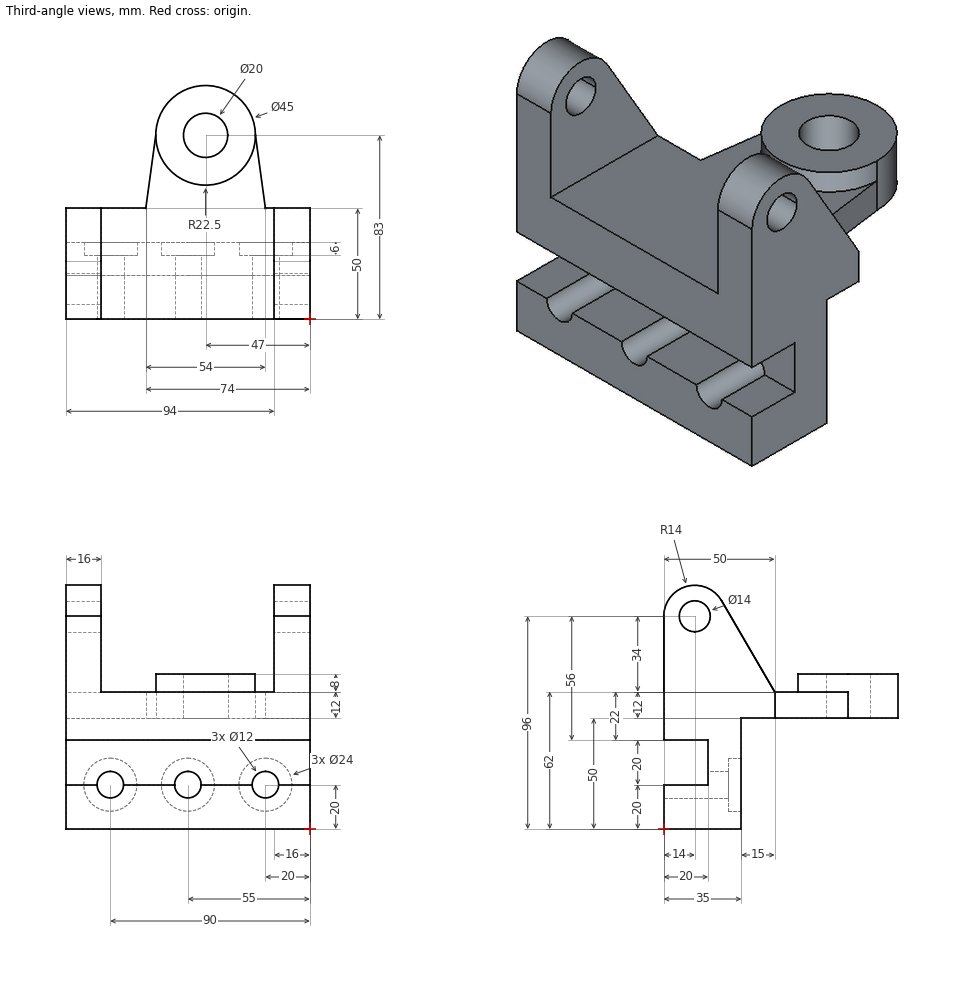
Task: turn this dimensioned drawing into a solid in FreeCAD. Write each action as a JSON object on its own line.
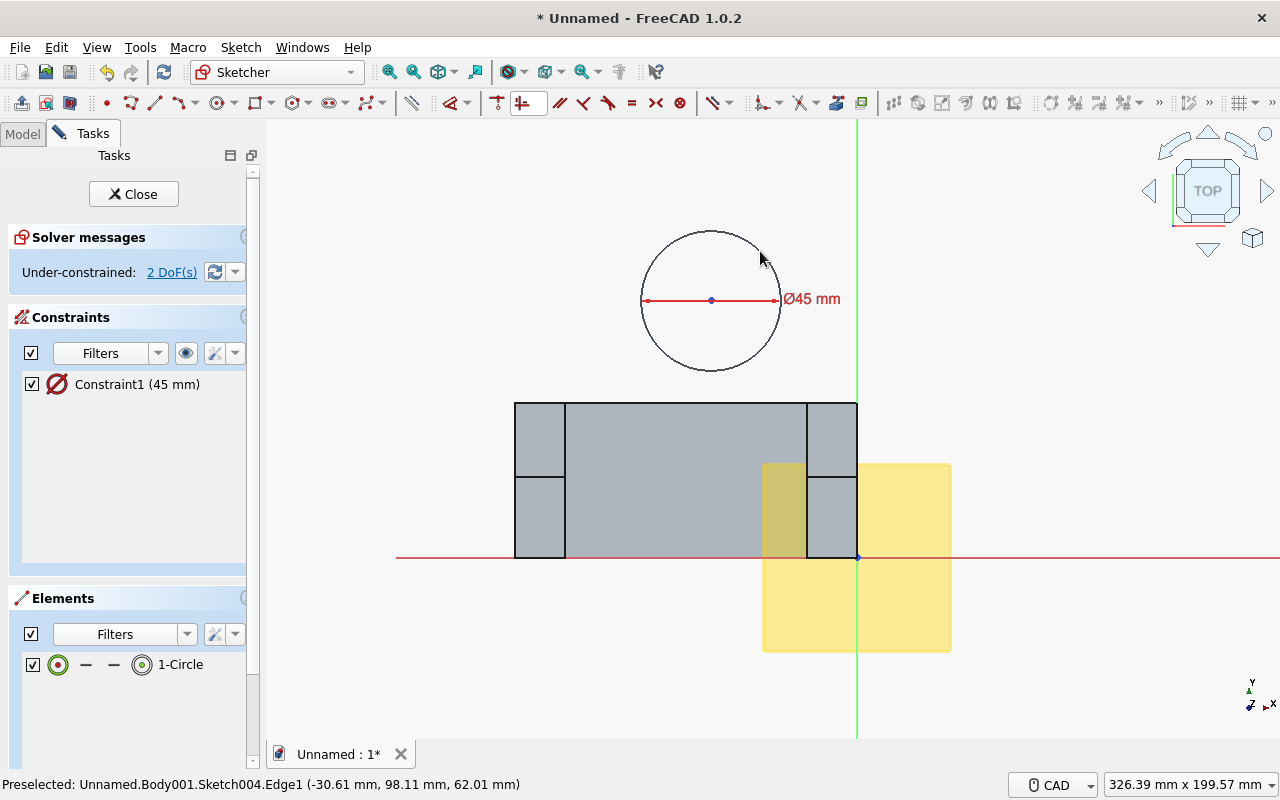
{"action": "left_click", "coordinate": [450, 104]}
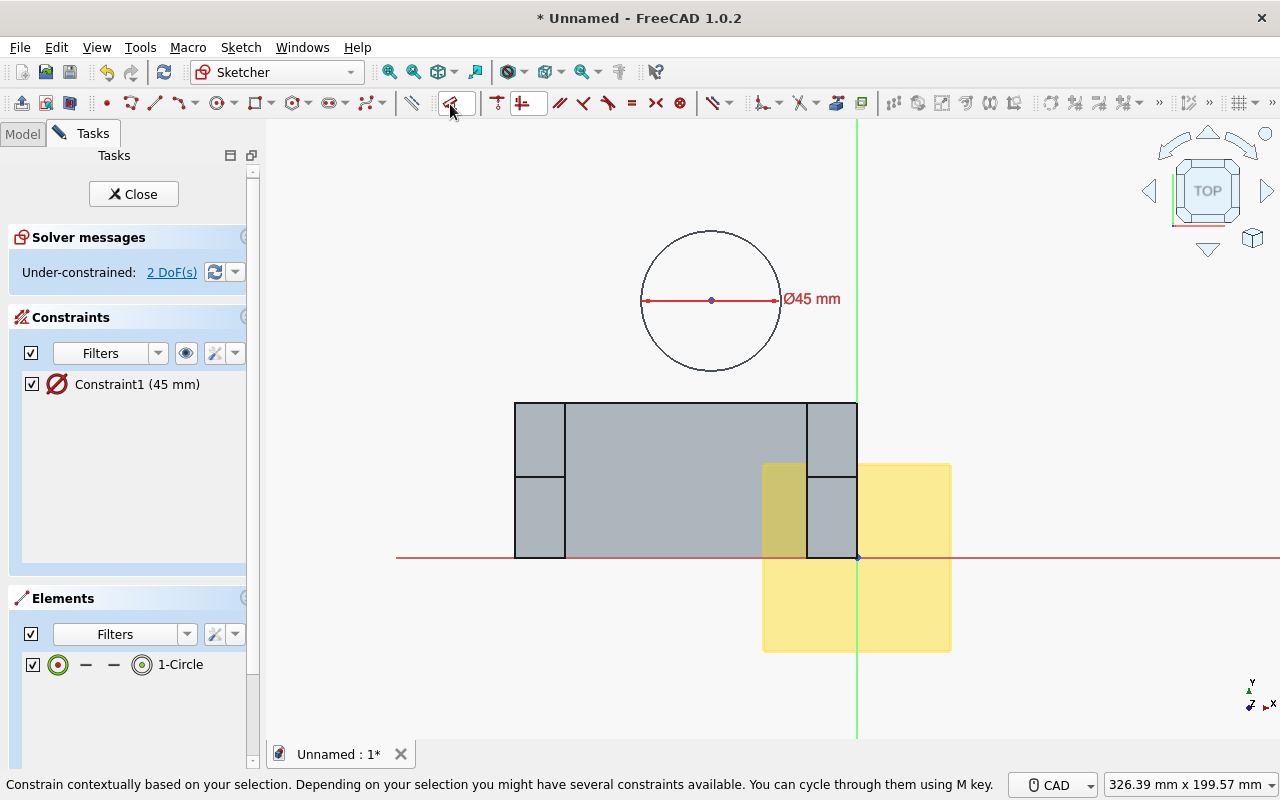
{"action": "left_click", "coordinate": [711, 301]}
{"action": "left_click", "coordinate": [784, 592]}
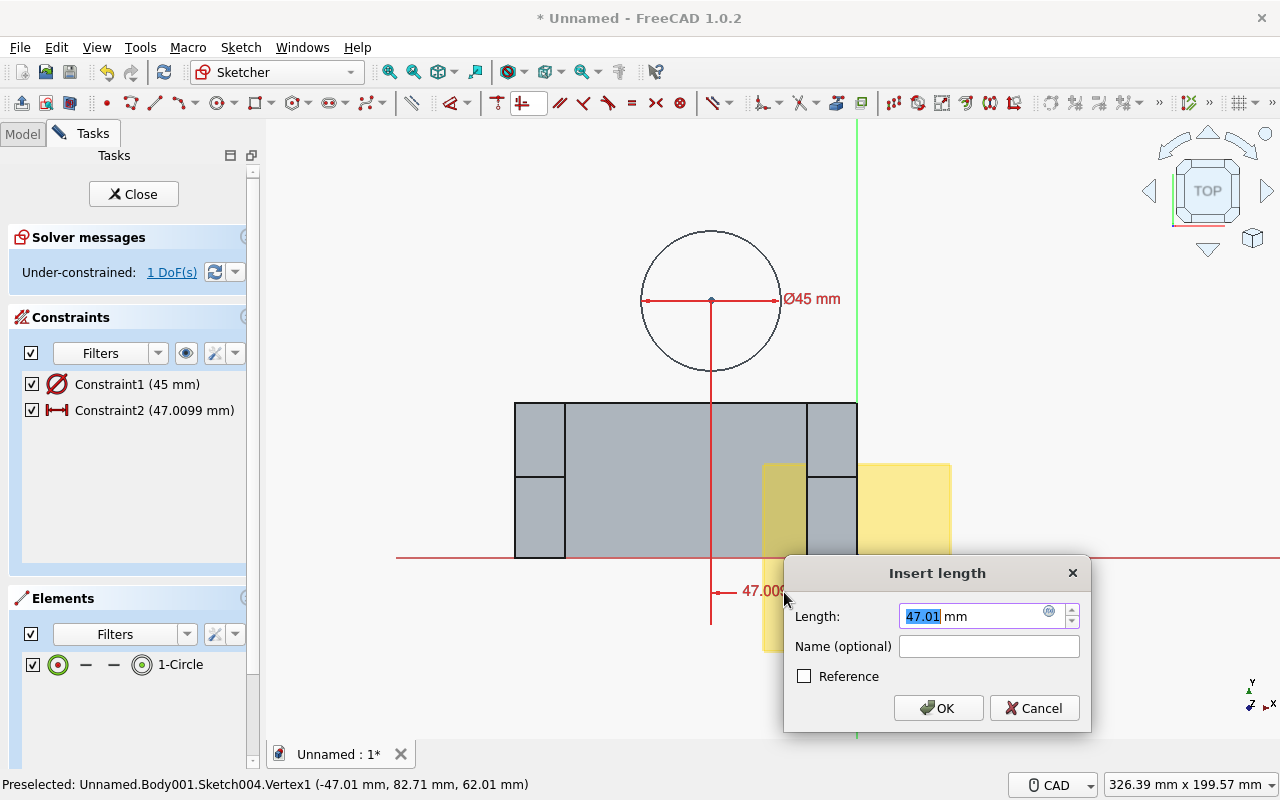
{"action": "type", "text": "47"}
{"action": "key", "text": "Return"}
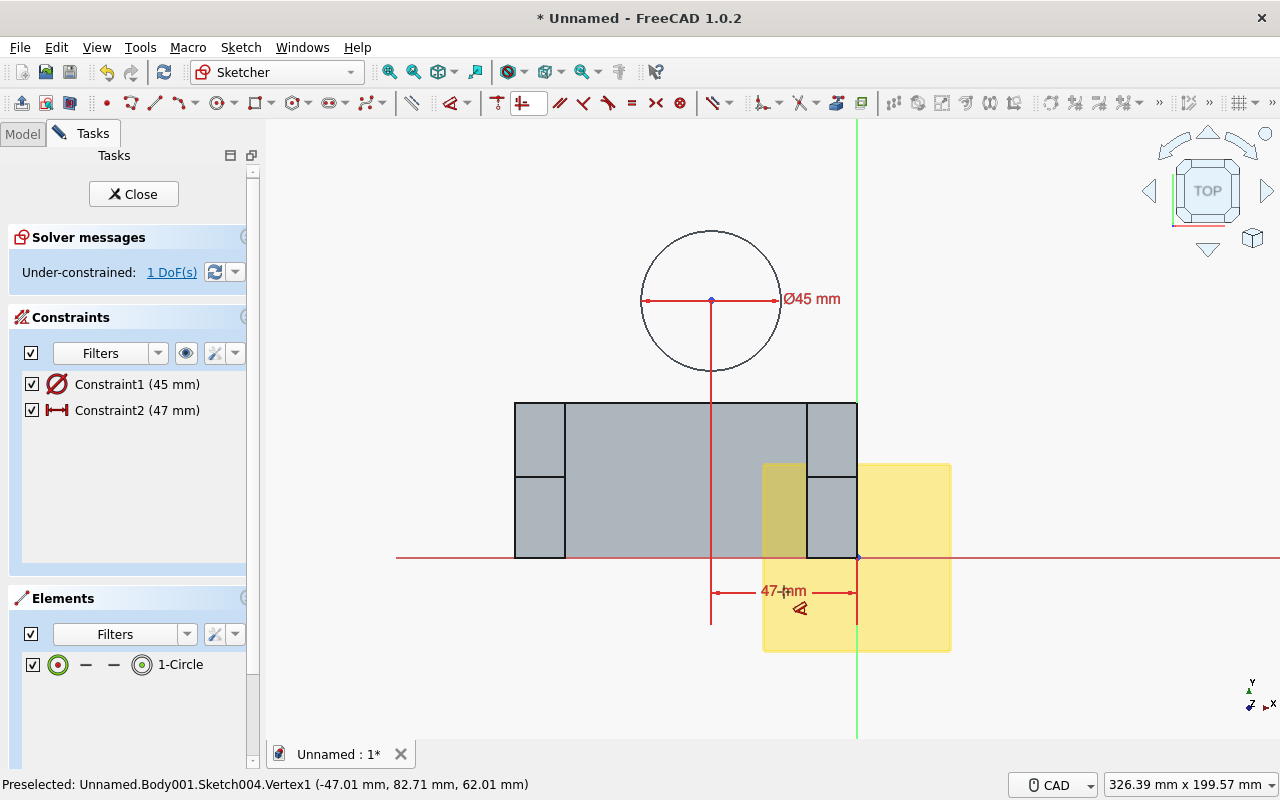
{"action": "left_click", "coordinate": [711, 301]}
{"action": "left_click", "coordinate": [891, 429]}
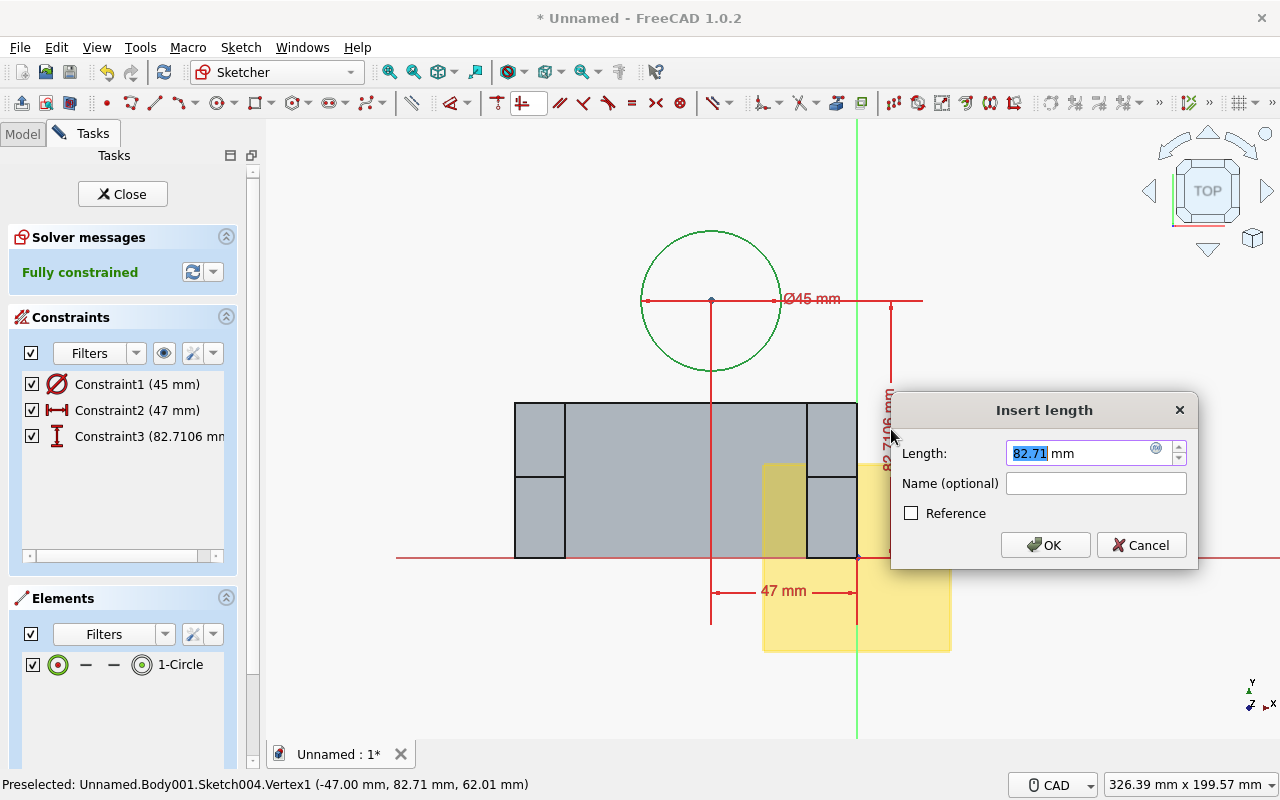
{"action": "type", "text": "83"}
{"action": "key", "text": "Return"}
{"action": "key", "text": "Escape"}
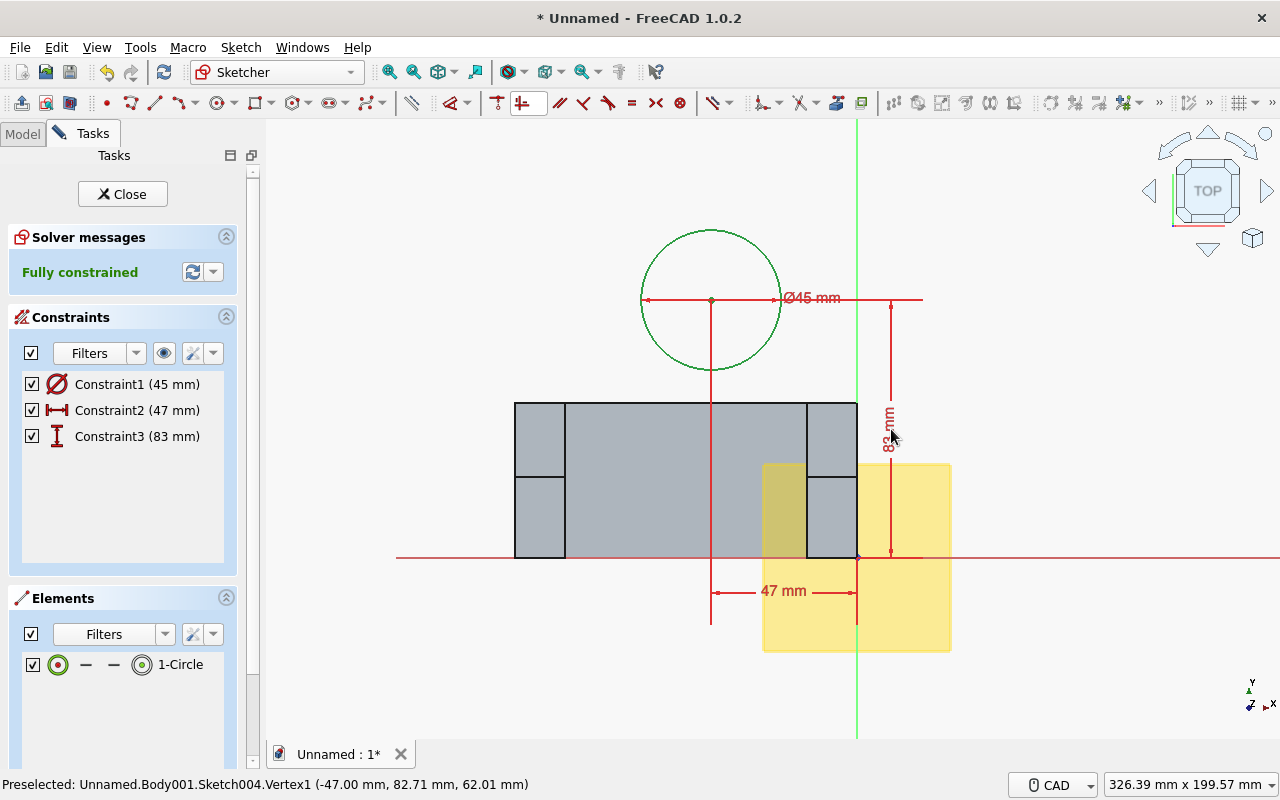
{"action": "left_click", "coordinate": [123, 194]}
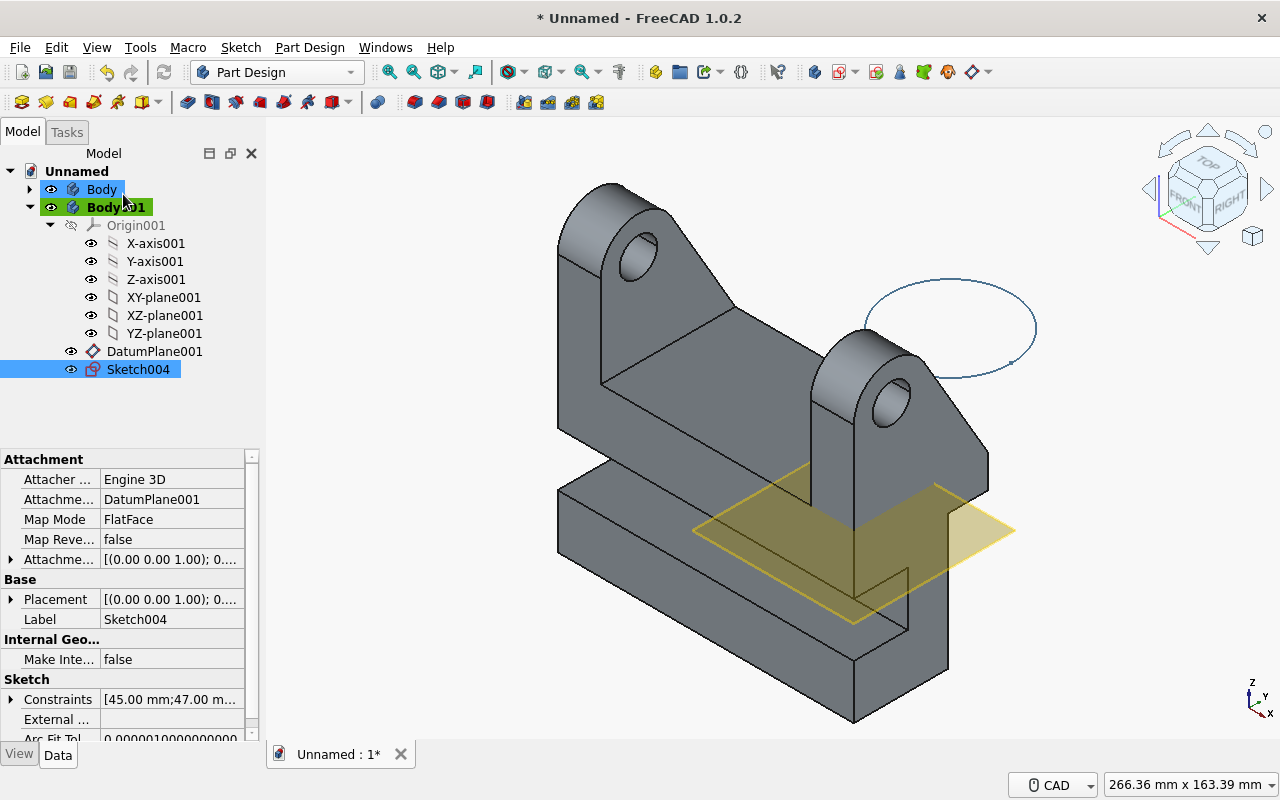
{"action": "left_click", "coordinate": [22, 102]}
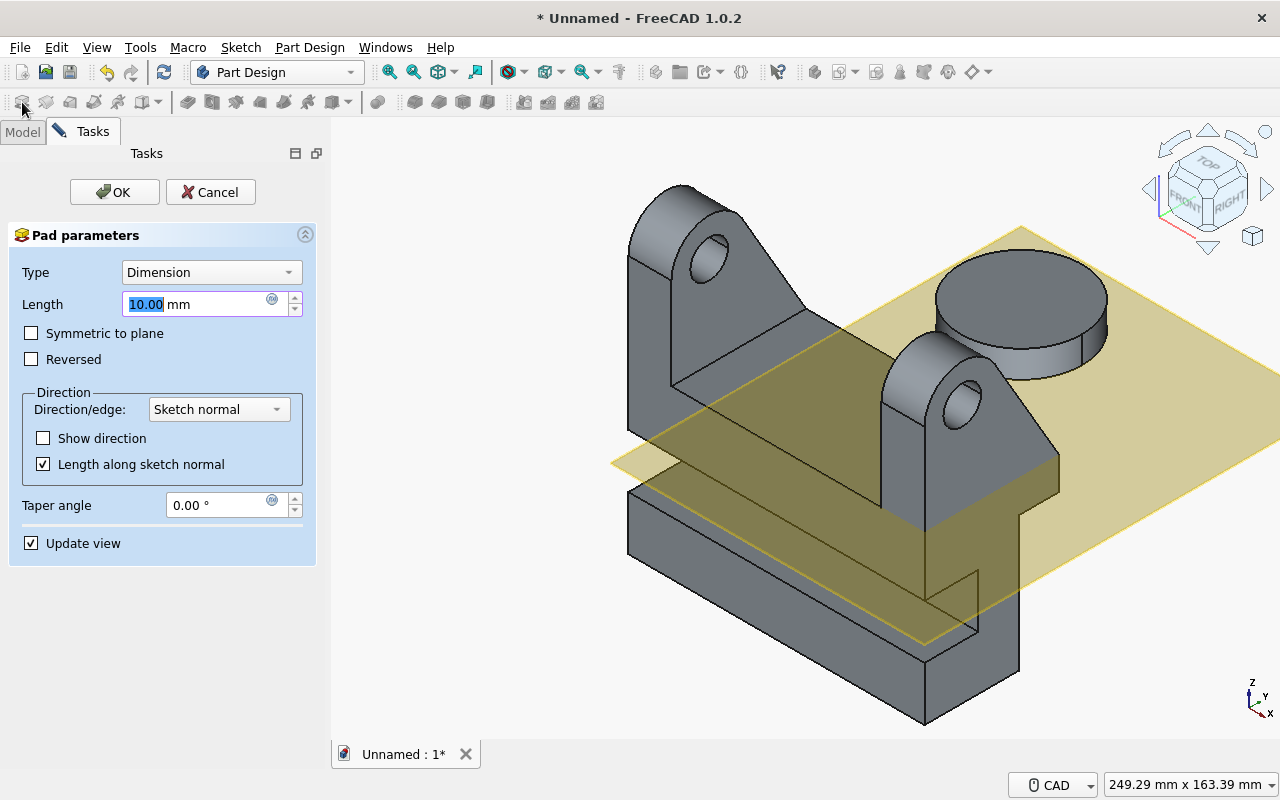
{"action": "left_click", "coordinate": [212, 272]}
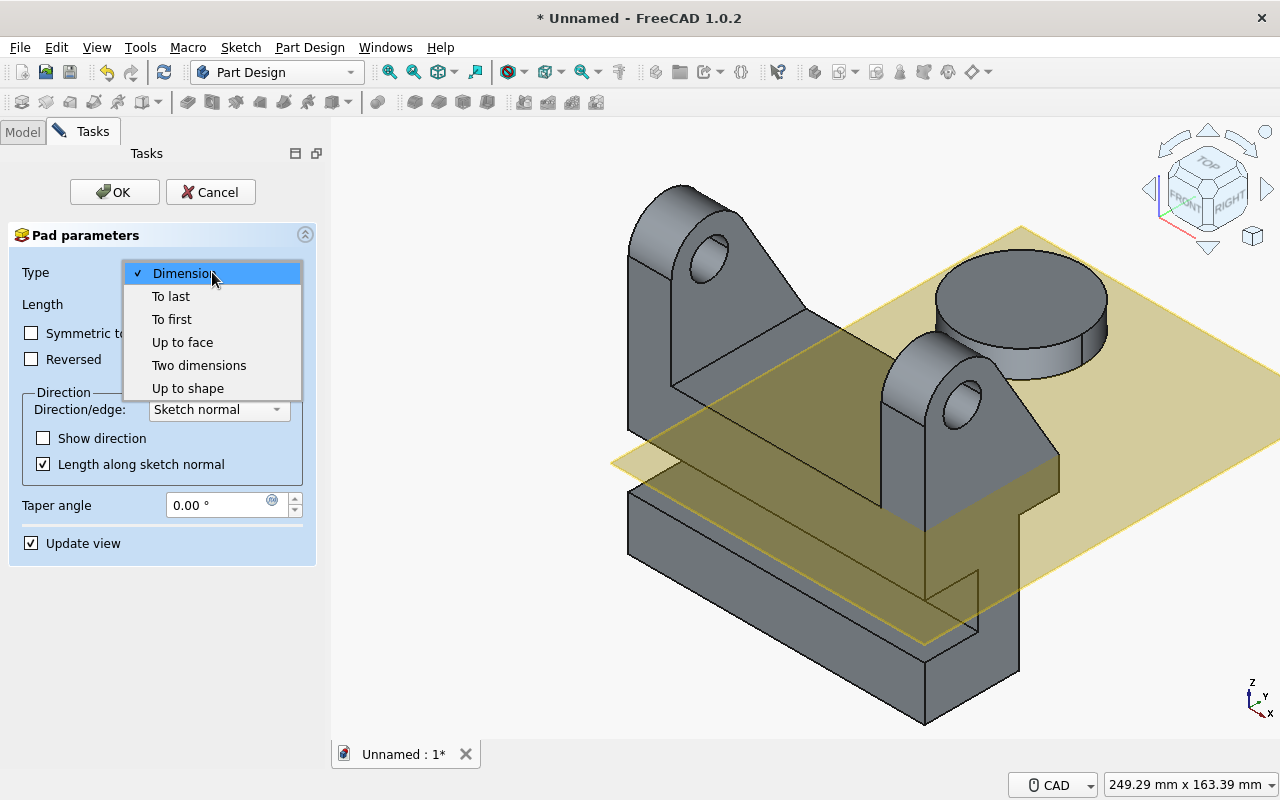
{"action": "left_click", "coordinate": [212, 366]}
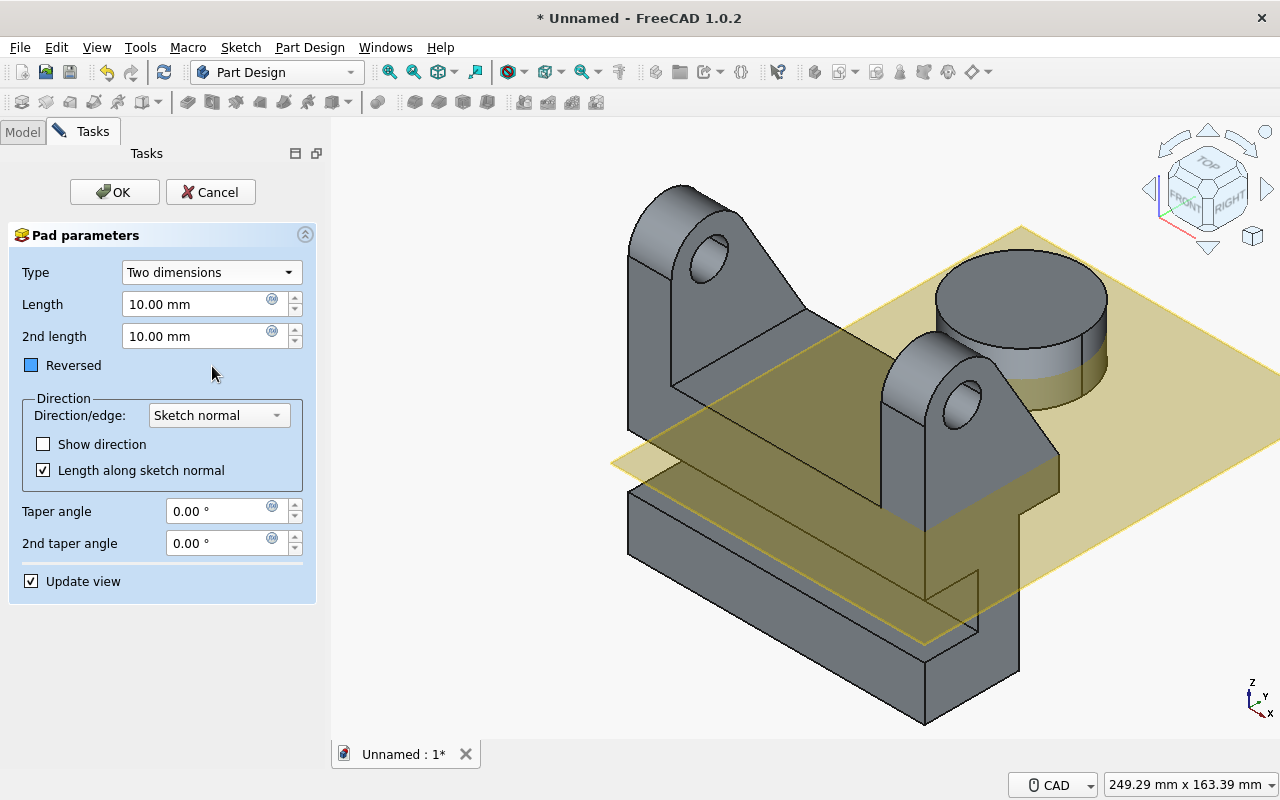
{"action": "triple_click", "coordinate": [204, 304]}